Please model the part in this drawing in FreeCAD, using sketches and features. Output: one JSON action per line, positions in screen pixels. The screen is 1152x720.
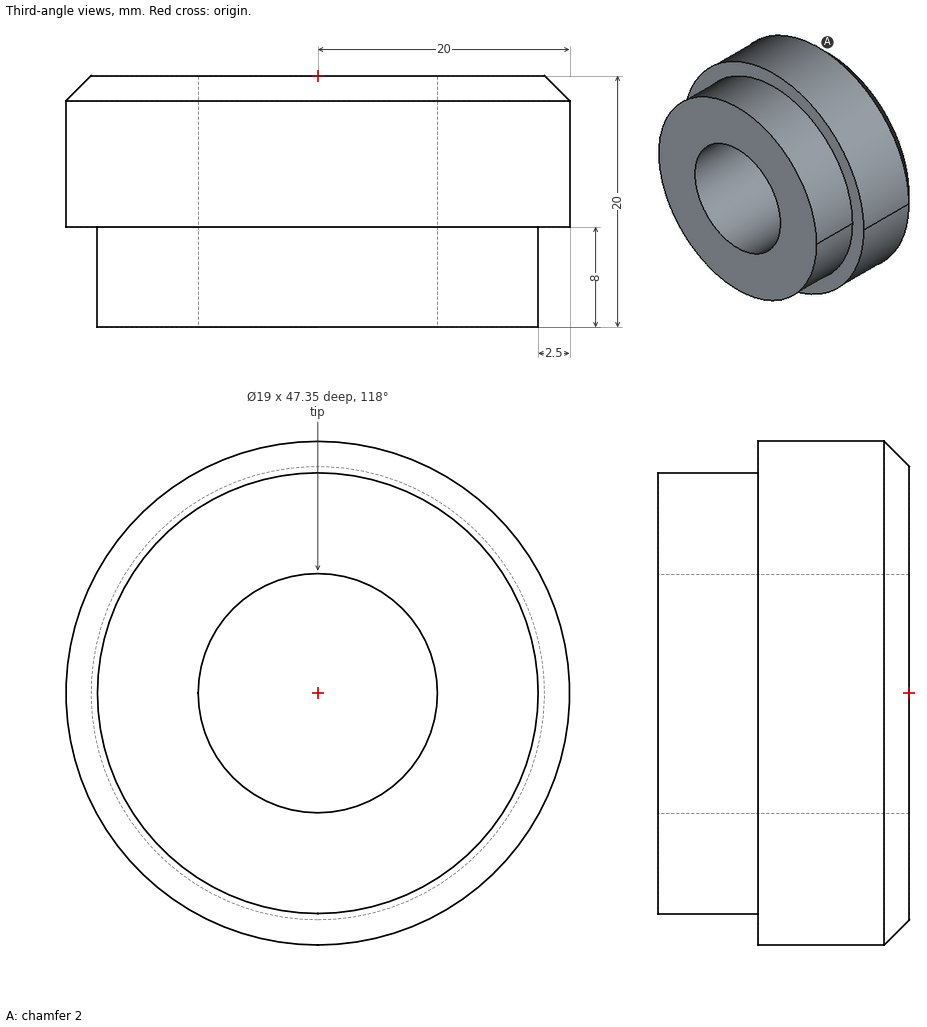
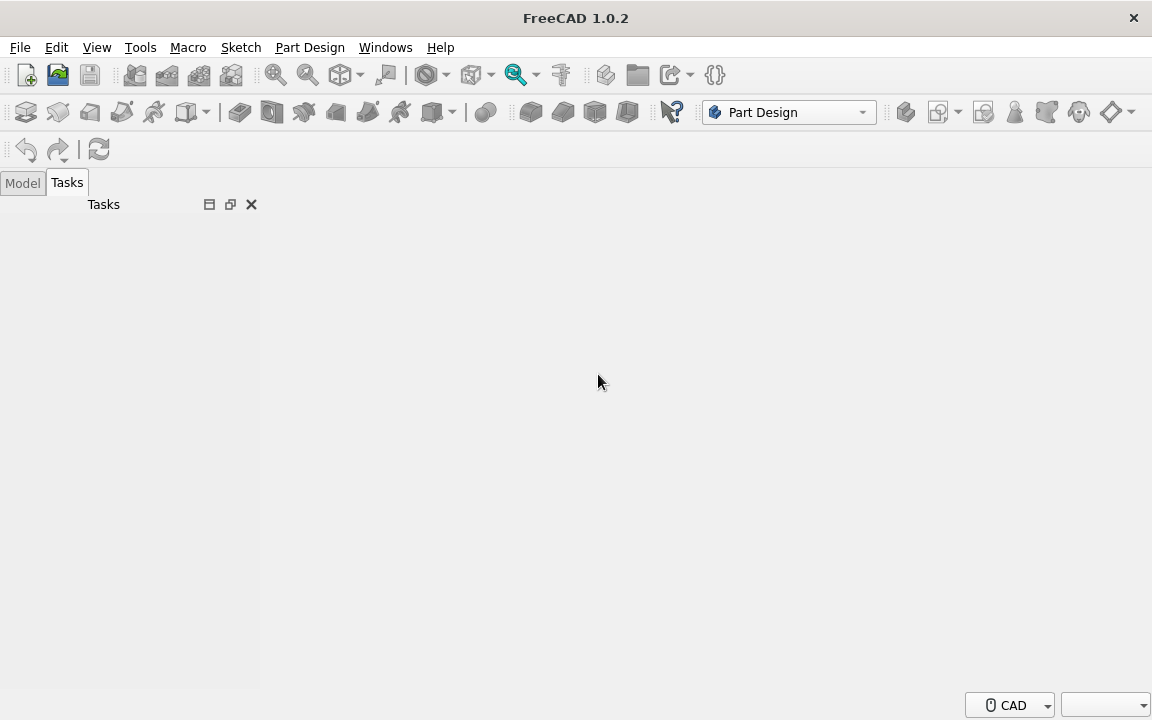
{"action": "left_click", "coordinate": [26, 76]}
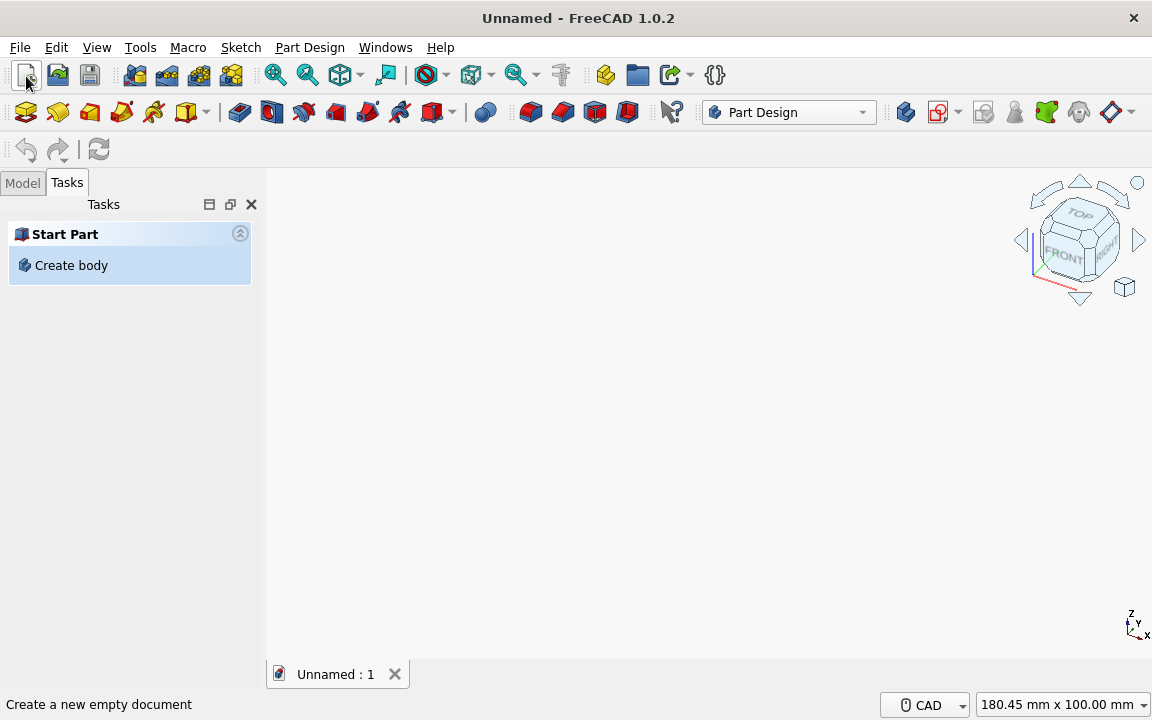
{"action": "left_click", "coordinate": [938, 112]}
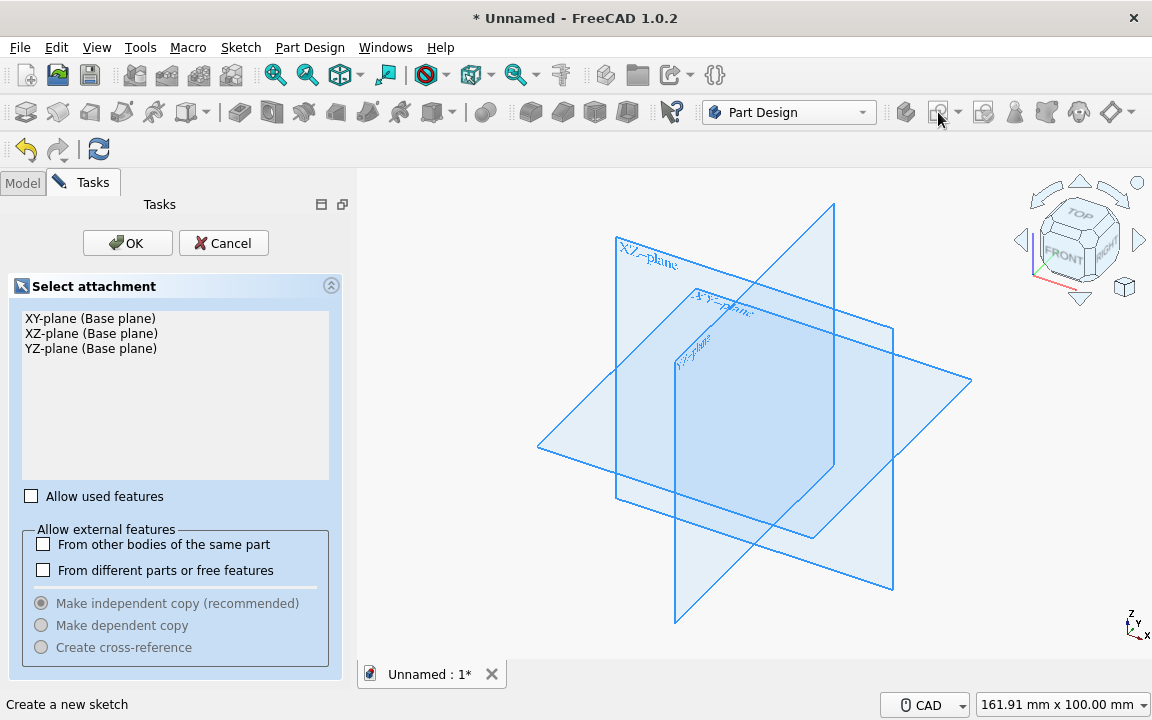
{"action": "left_click", "coordinate": [82, 318]}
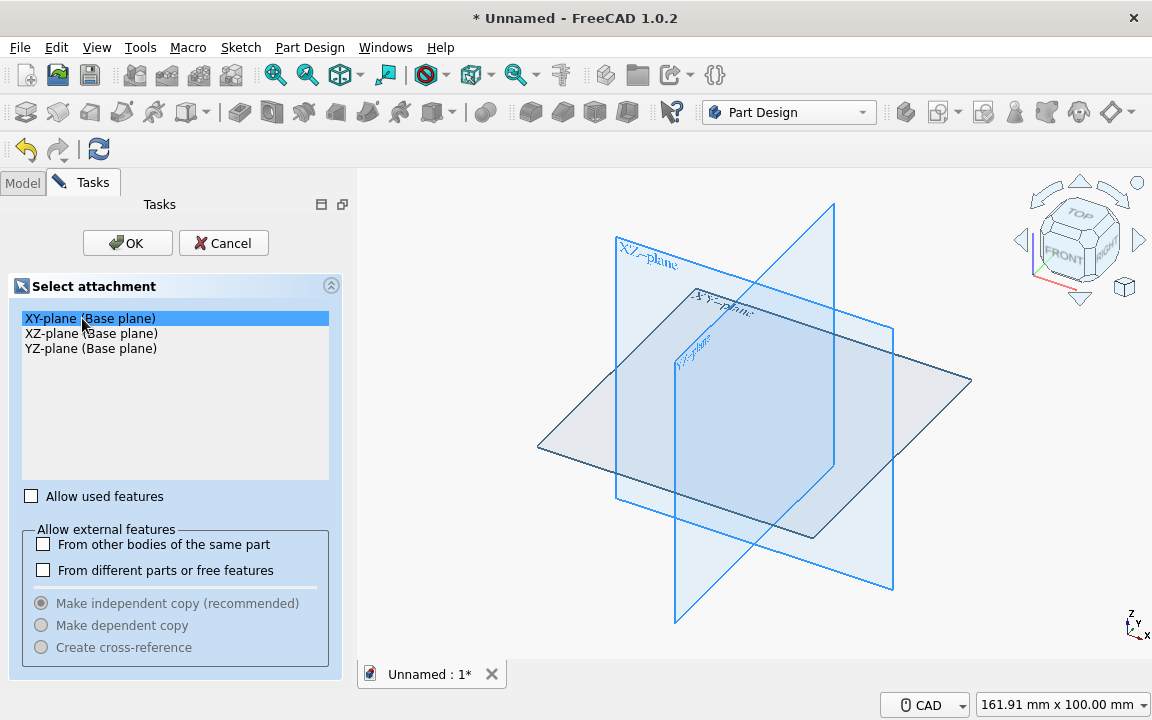
{"action": "left_click", "coordinate": [128, 243]}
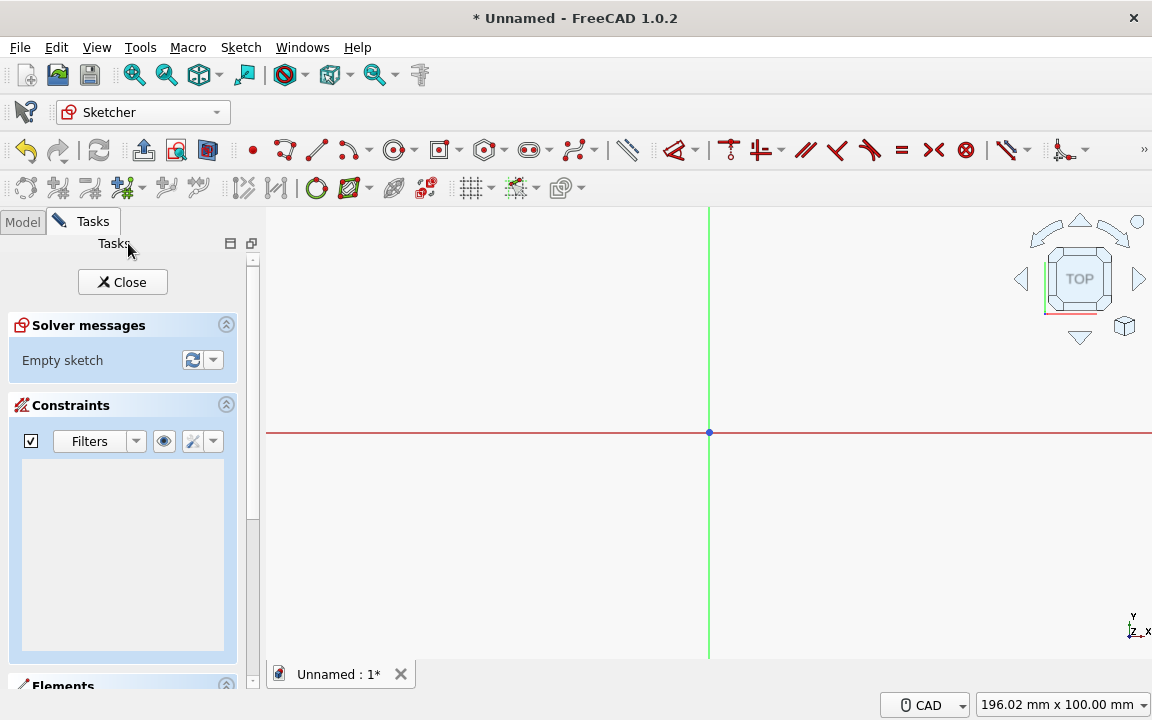
{"action": "scroll", "coordinate": [803, 498], "scroll_direction": "up", "scroll_amount": 6}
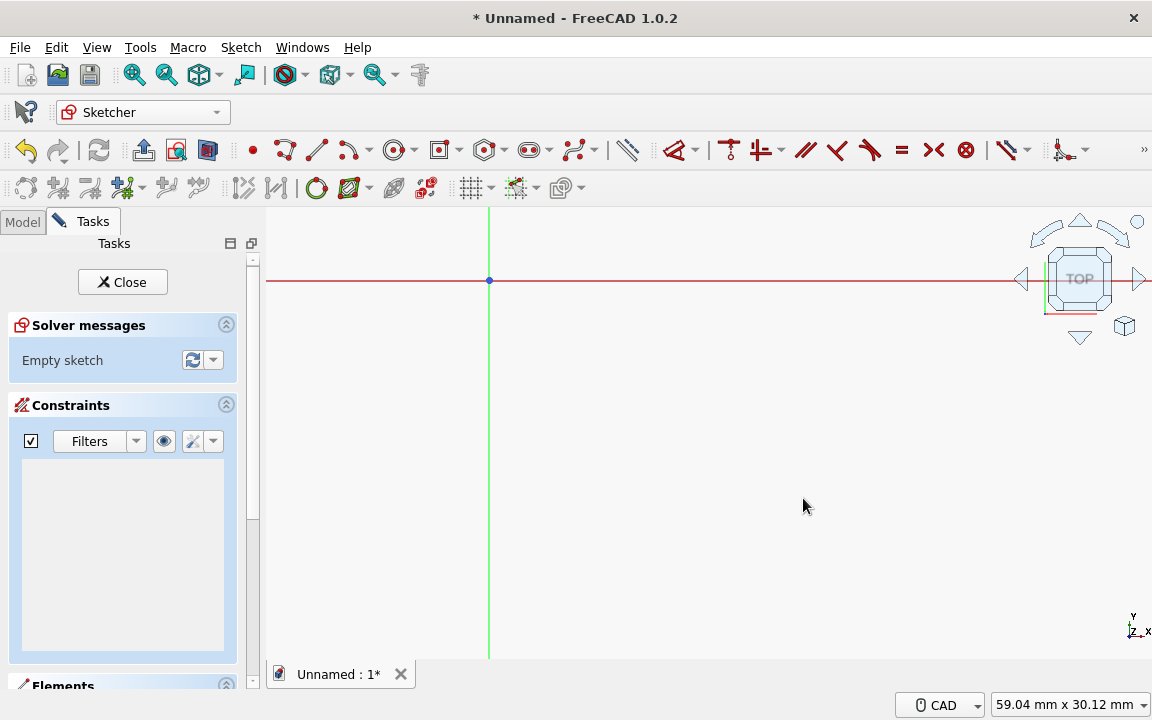
{"action": "left_click", "coordinate": [286, 150]}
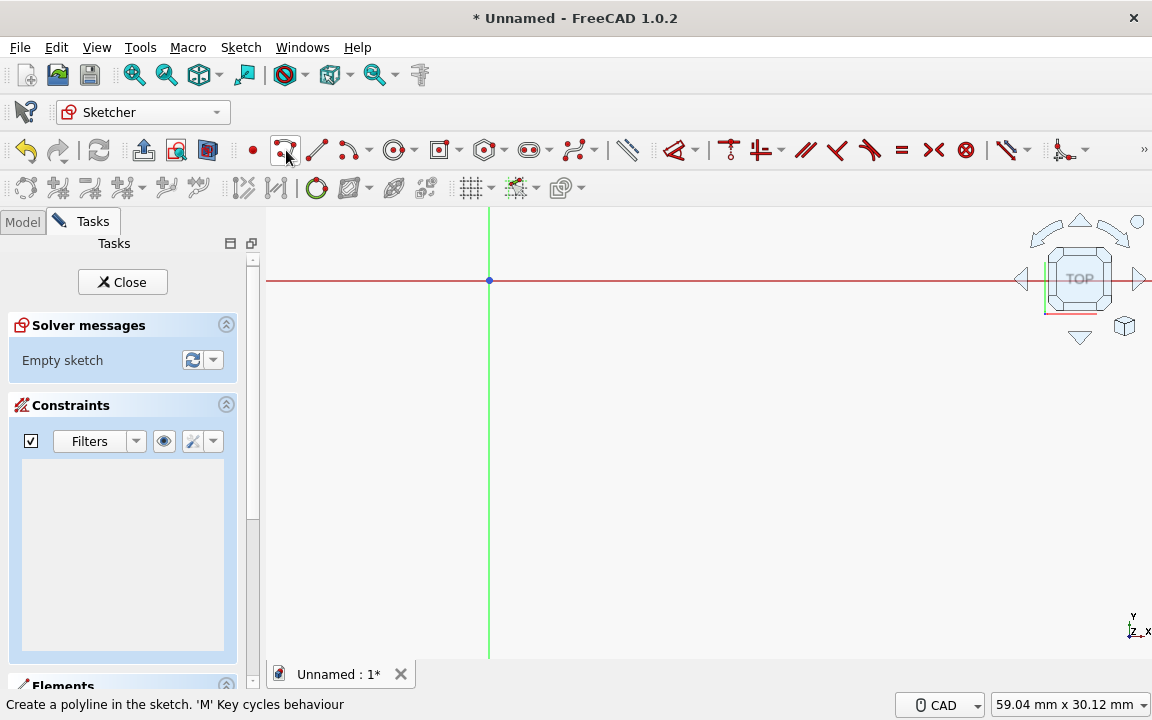
{"action": "left_click", "coordinate": [490, 281]}
{"action": "left_click", "coordinate": [499, 581]}
{"action": "left_click", "coordinate": [752, 581]}
{"action": "left_click", "coordinate": [752, 461]}
{"action": "left_click", "coordinate": [790, 461]}
{"action": "left_click", "coordinate": [790, 290]}
{"action": "left_click", "coordinate": [490, 281]}
{"action": "key", "text": "Escape"}
{"action": "key", "text": "Escape"}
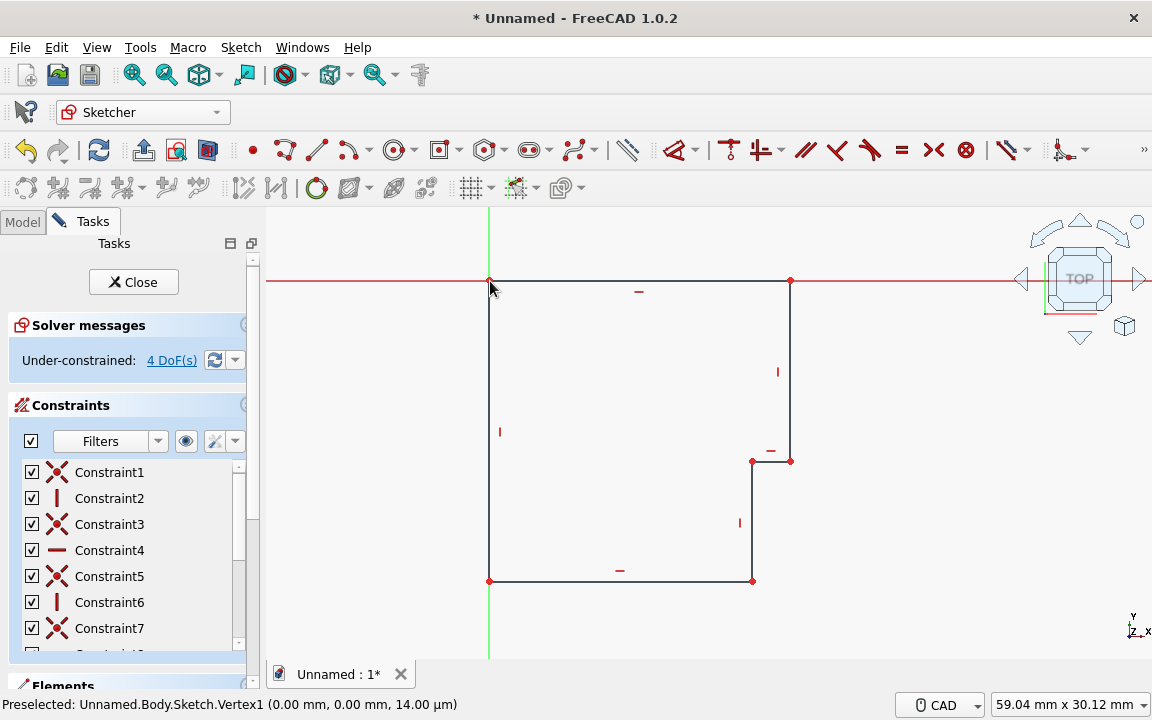
{"action": "left_click", "coordinate": [752, 546]}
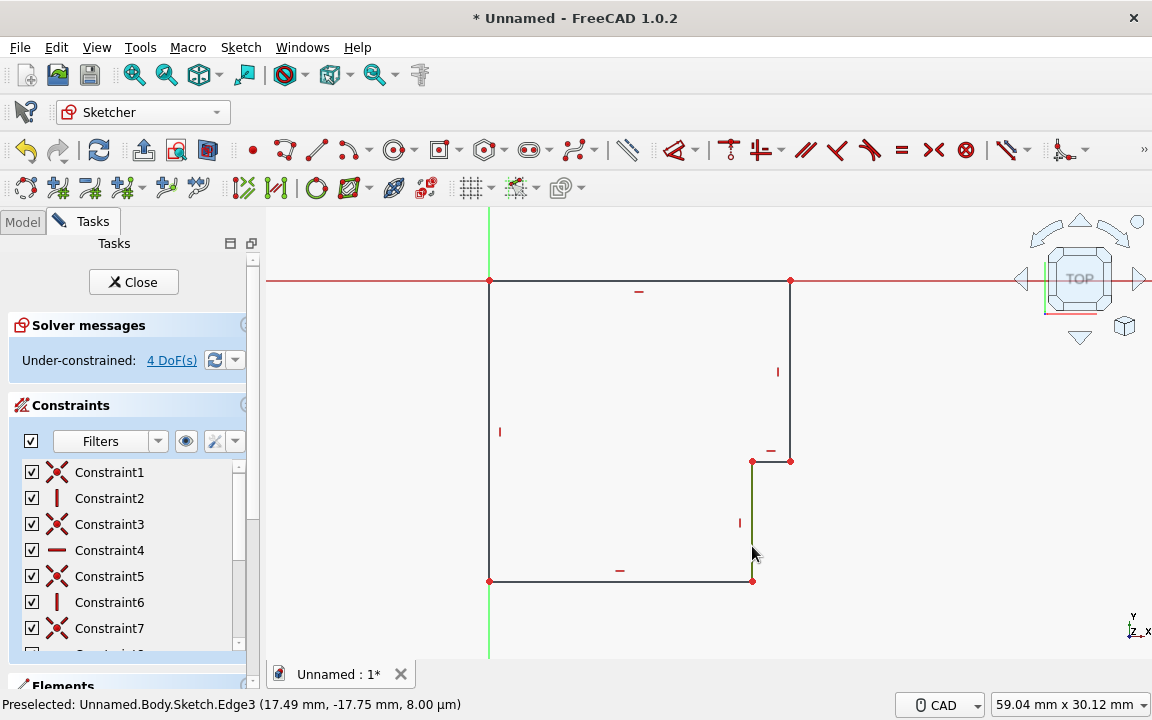
{"action": "key", "text": "i"}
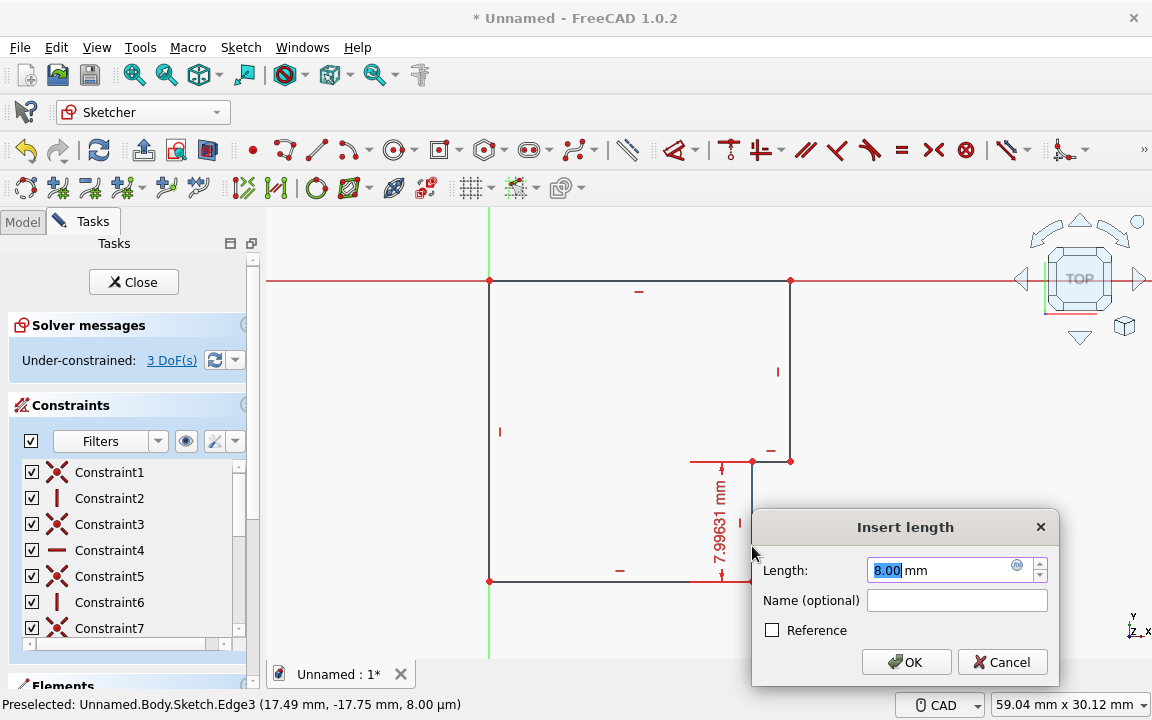
{"action": "type", "text": "8"}
{"action": "key", "text": "Return"}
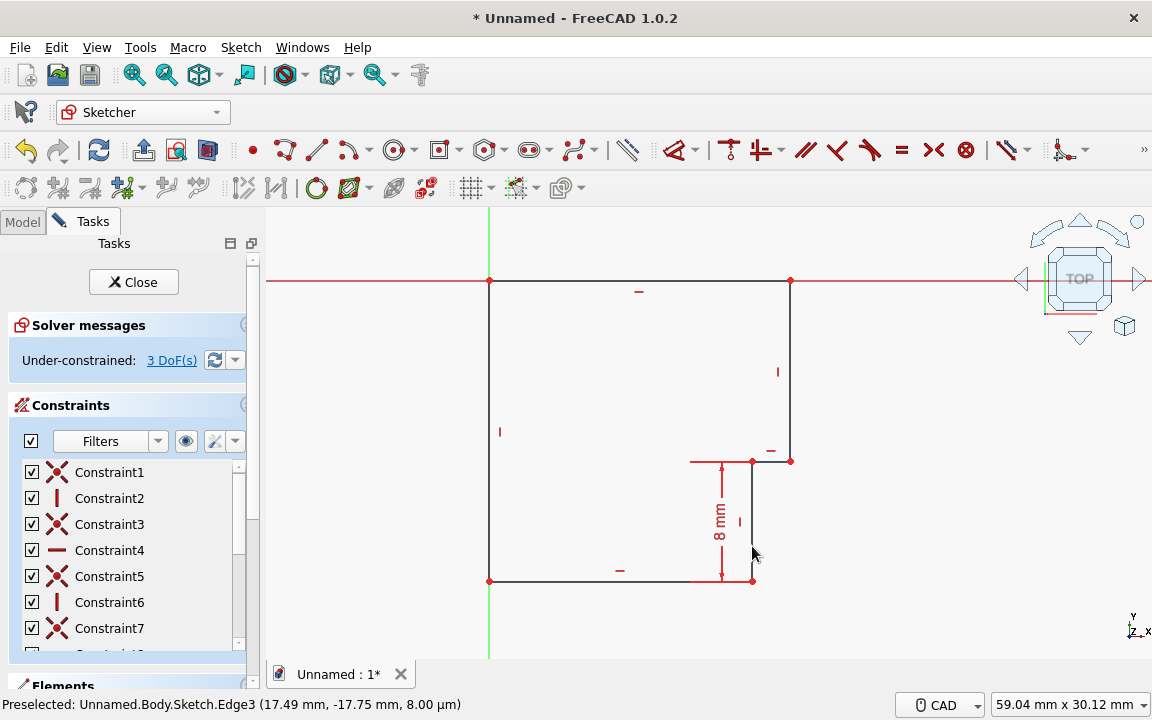
{"action": "left_click", "coordinate": [490, 371]}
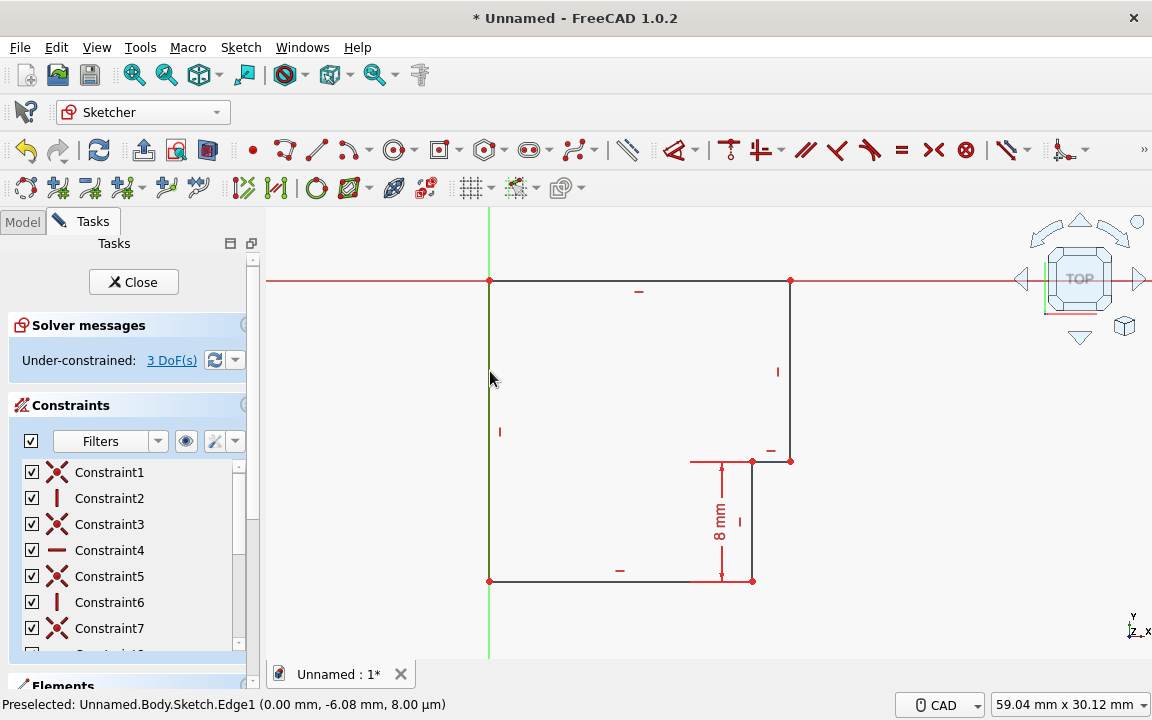
{"action": "key", "text": "i"}